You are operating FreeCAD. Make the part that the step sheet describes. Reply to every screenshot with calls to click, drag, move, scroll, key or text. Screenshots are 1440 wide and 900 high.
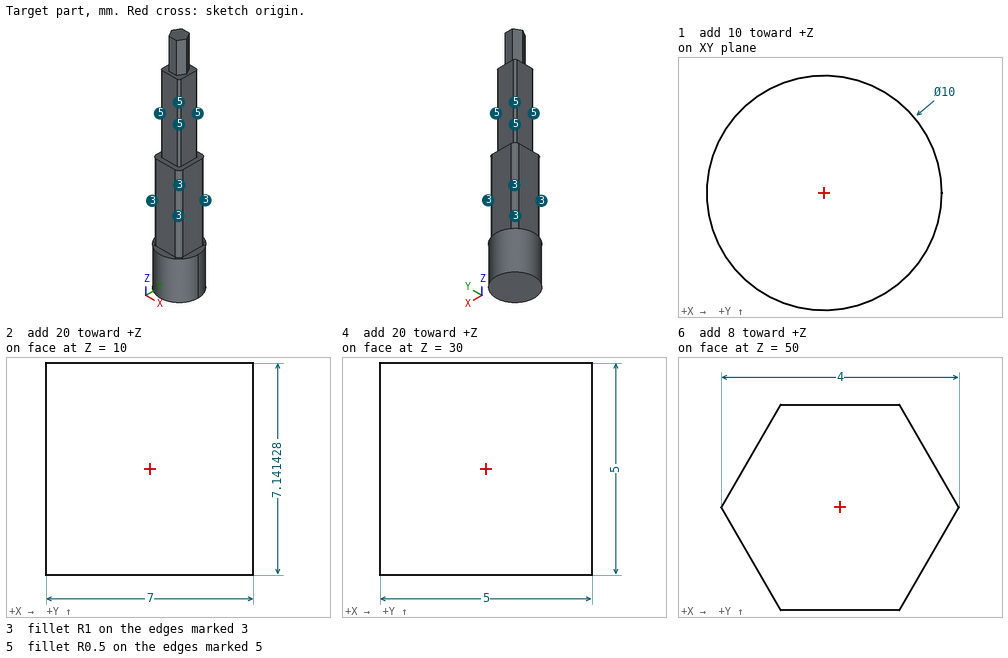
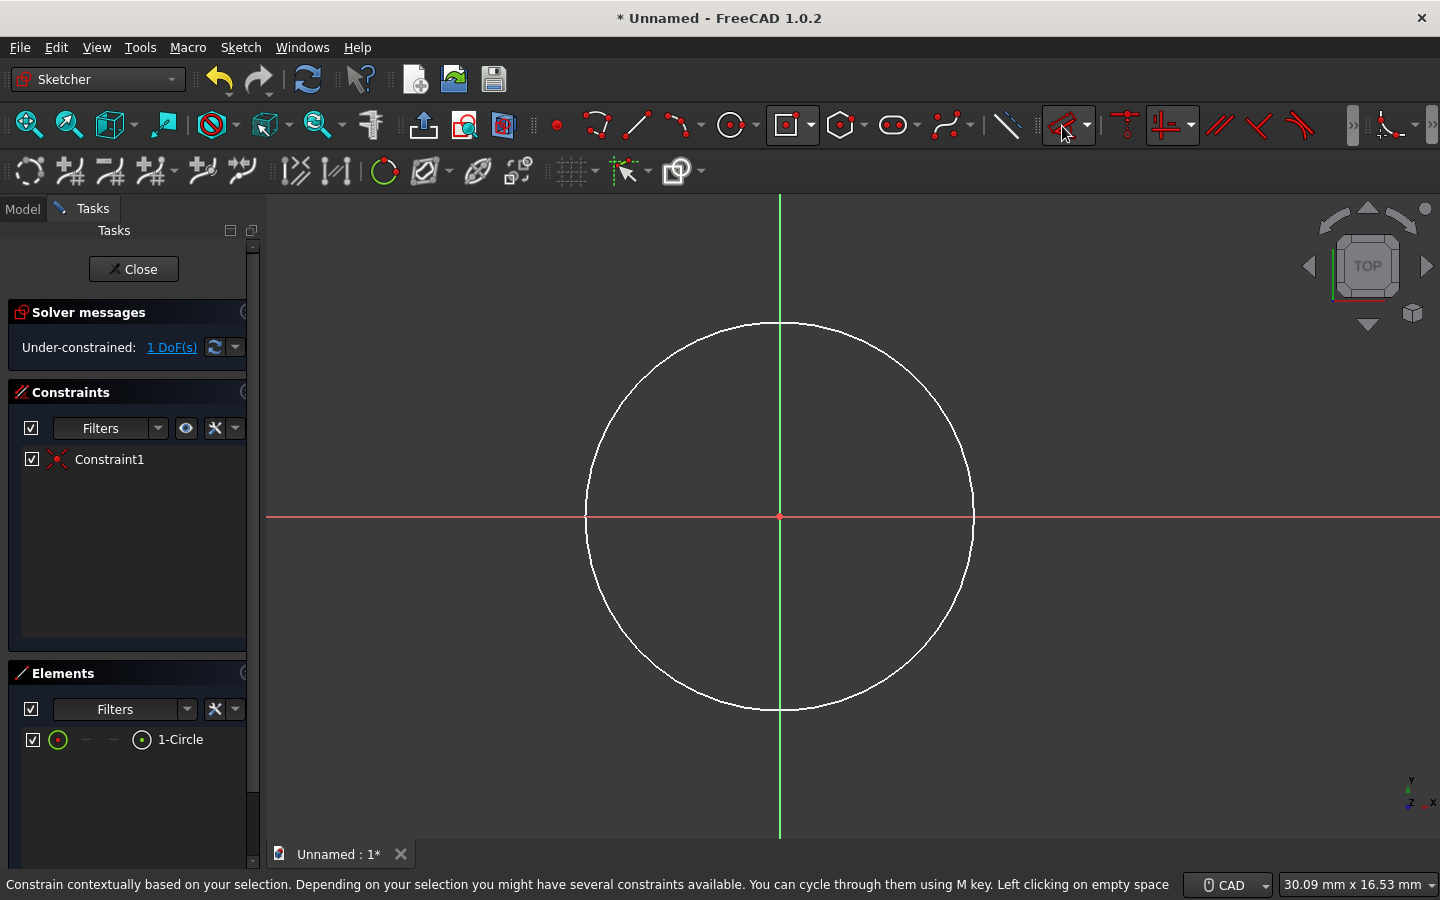
click(917, 379)
click(940, 356)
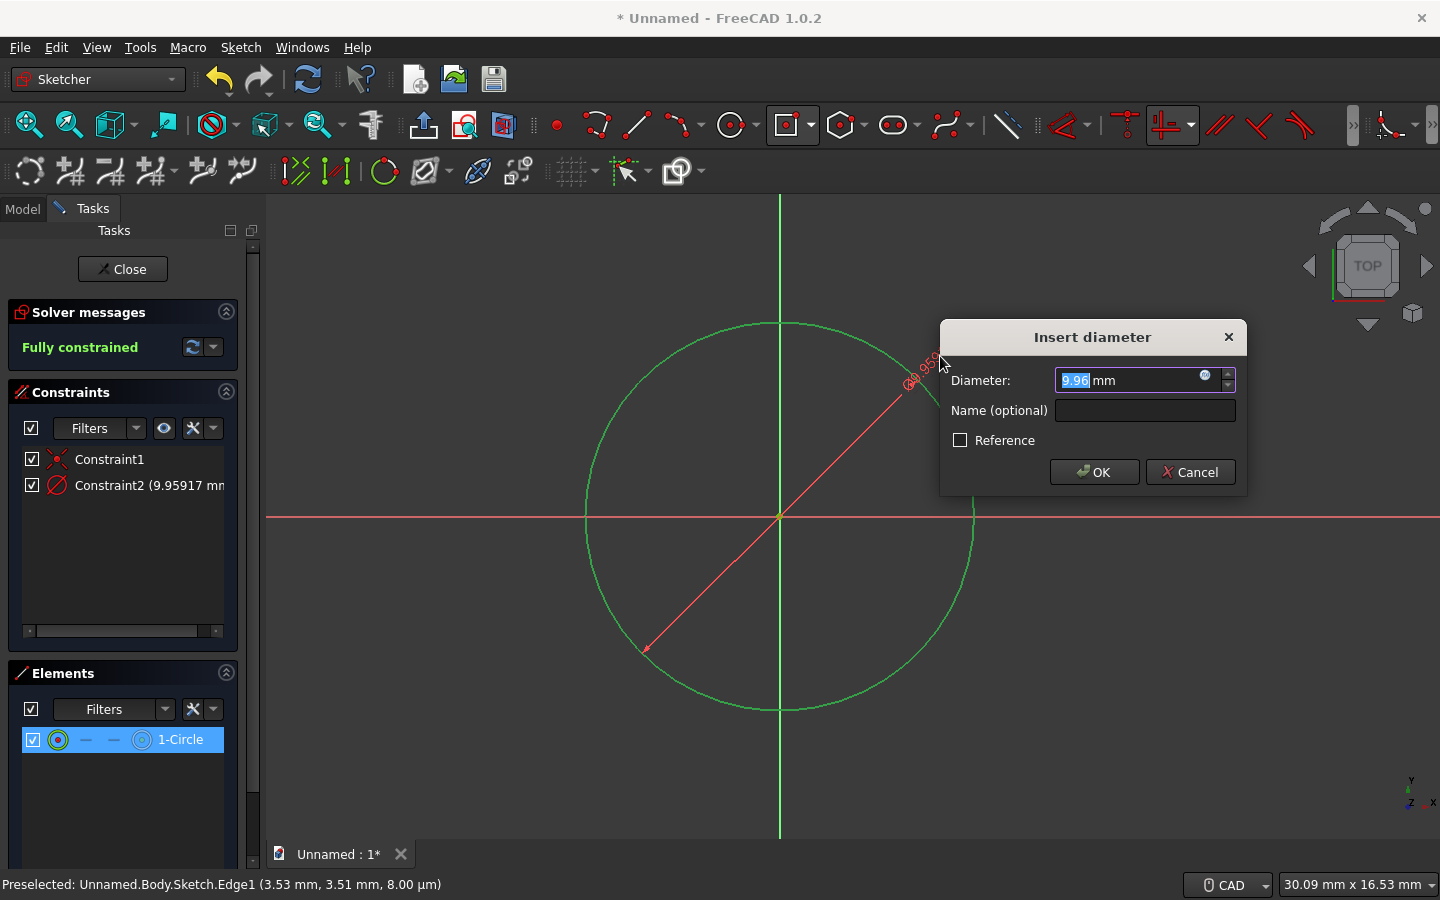
text(10)
key(Return)
key(Escape)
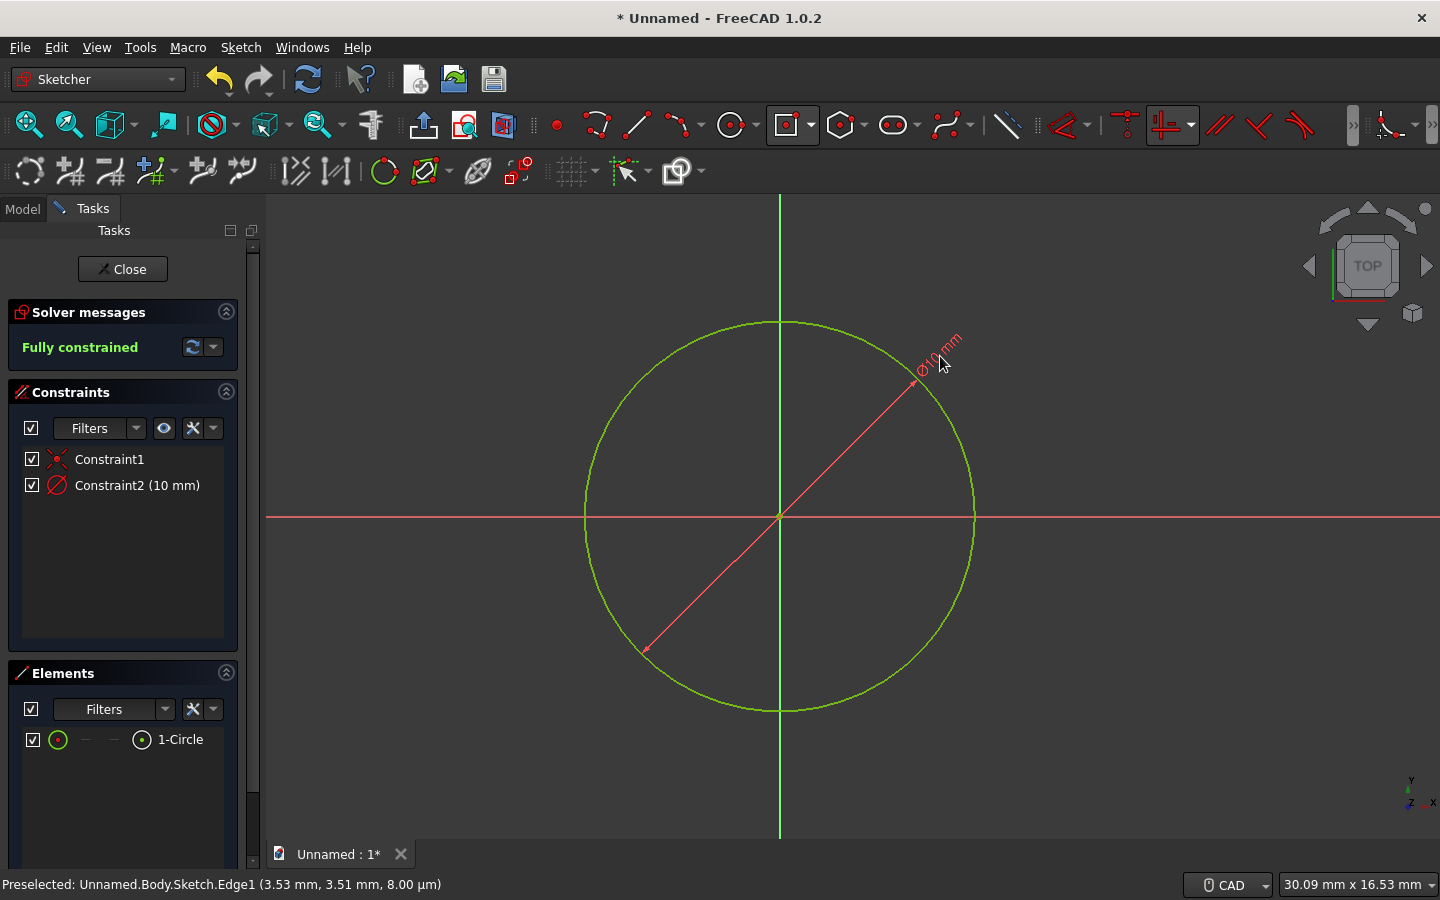
click(123, 269)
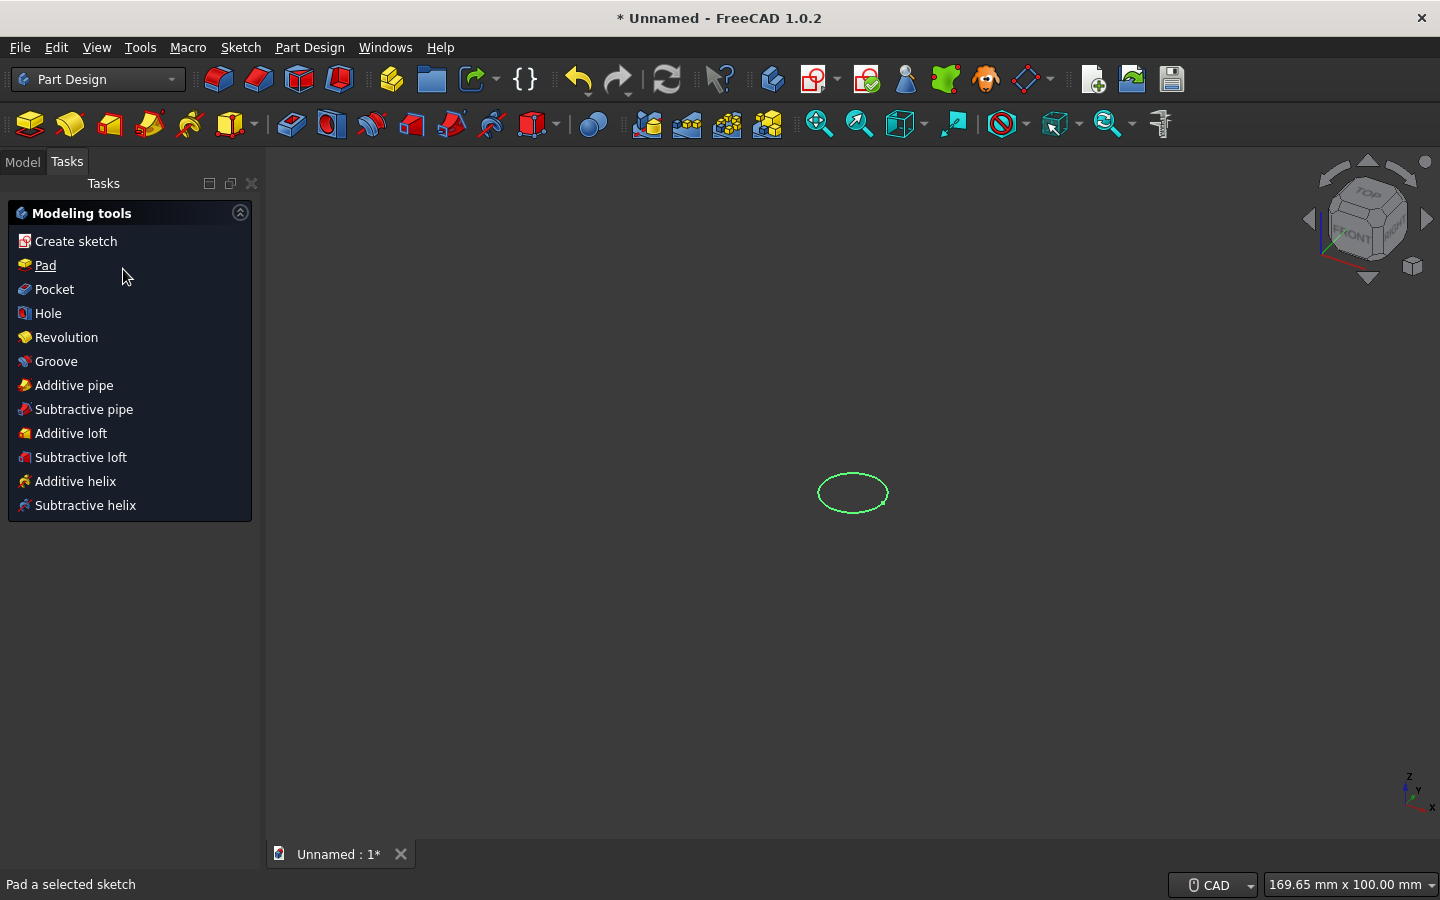
click(30, 124)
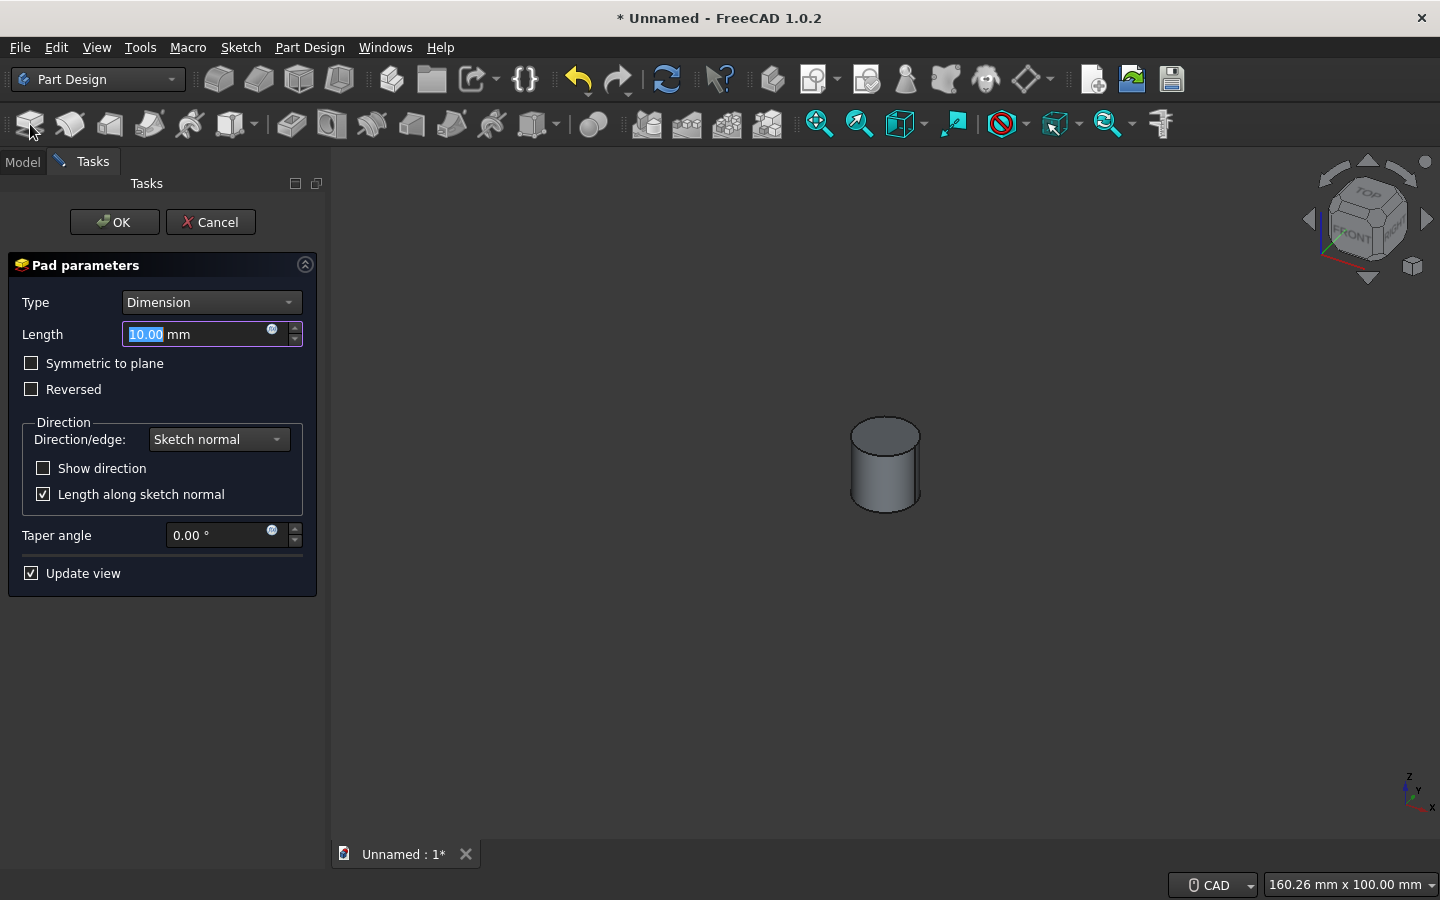
text(10)
key(Tab)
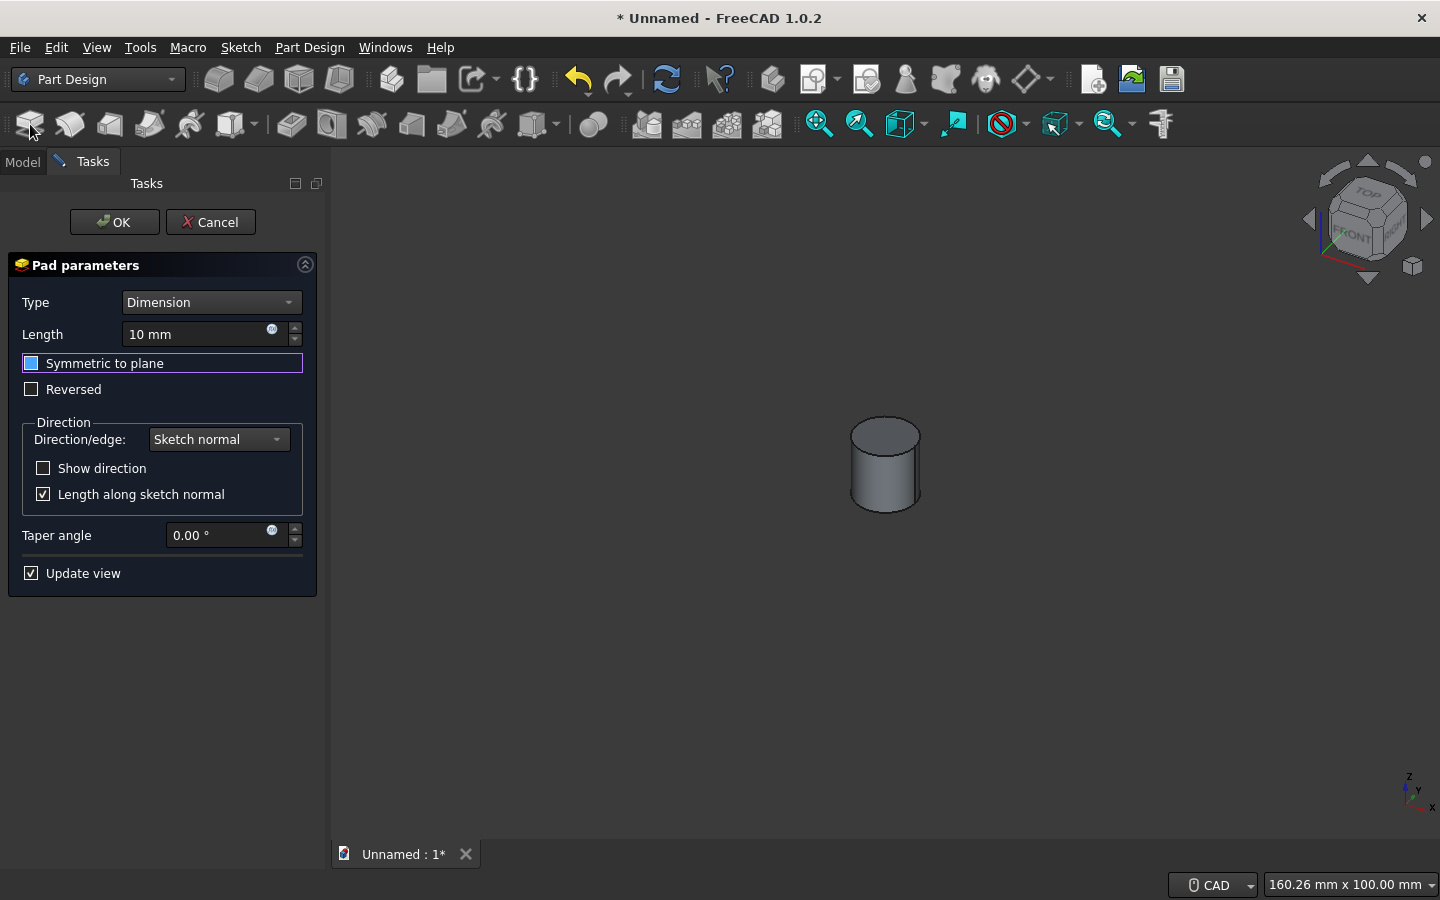
click(115, 222)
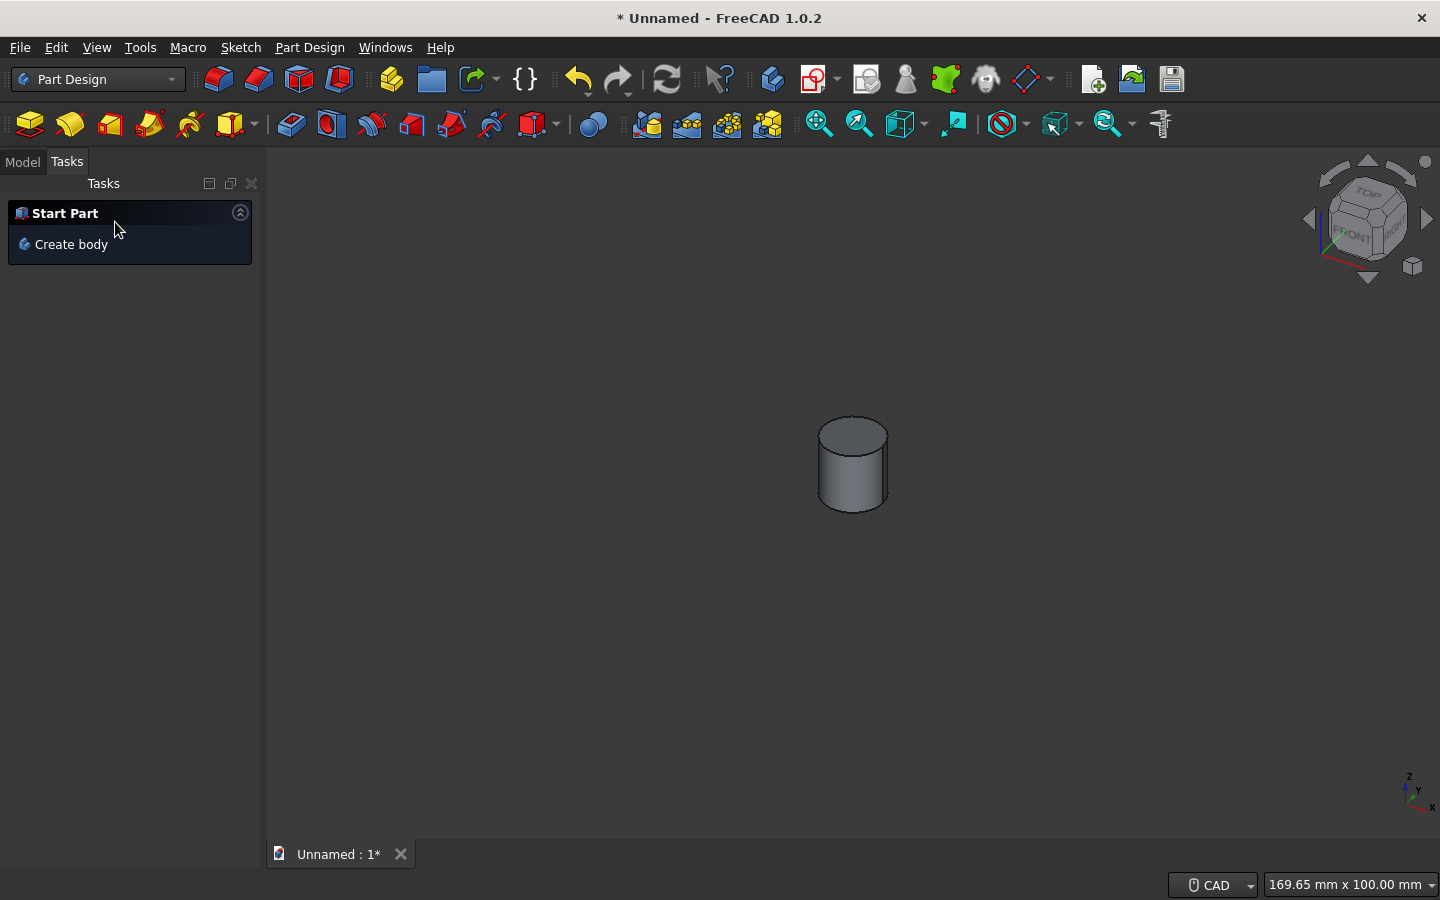
click(820, 124)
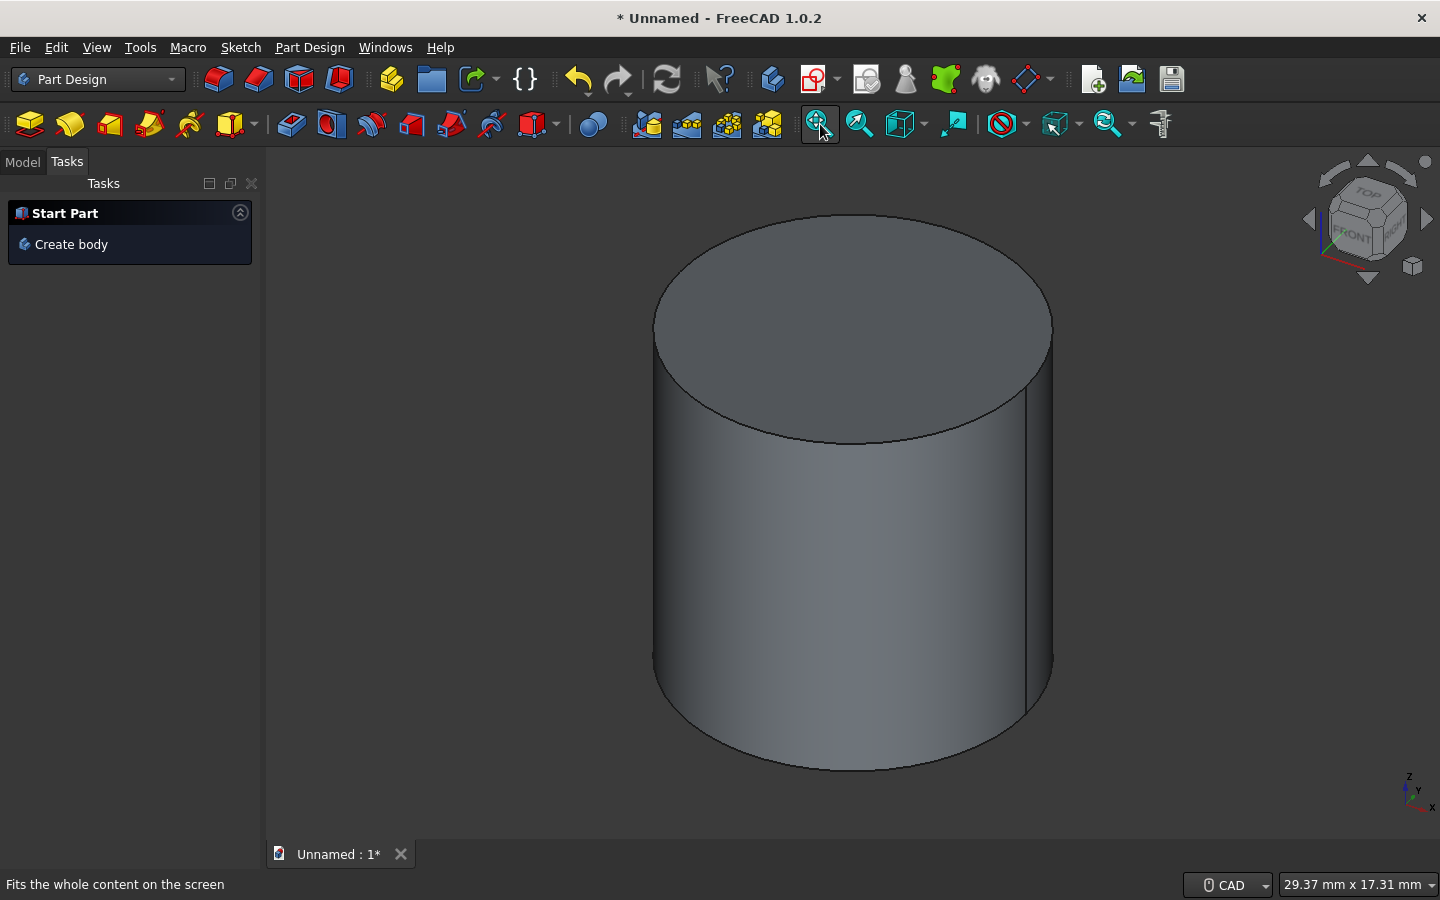
click(853, 328)